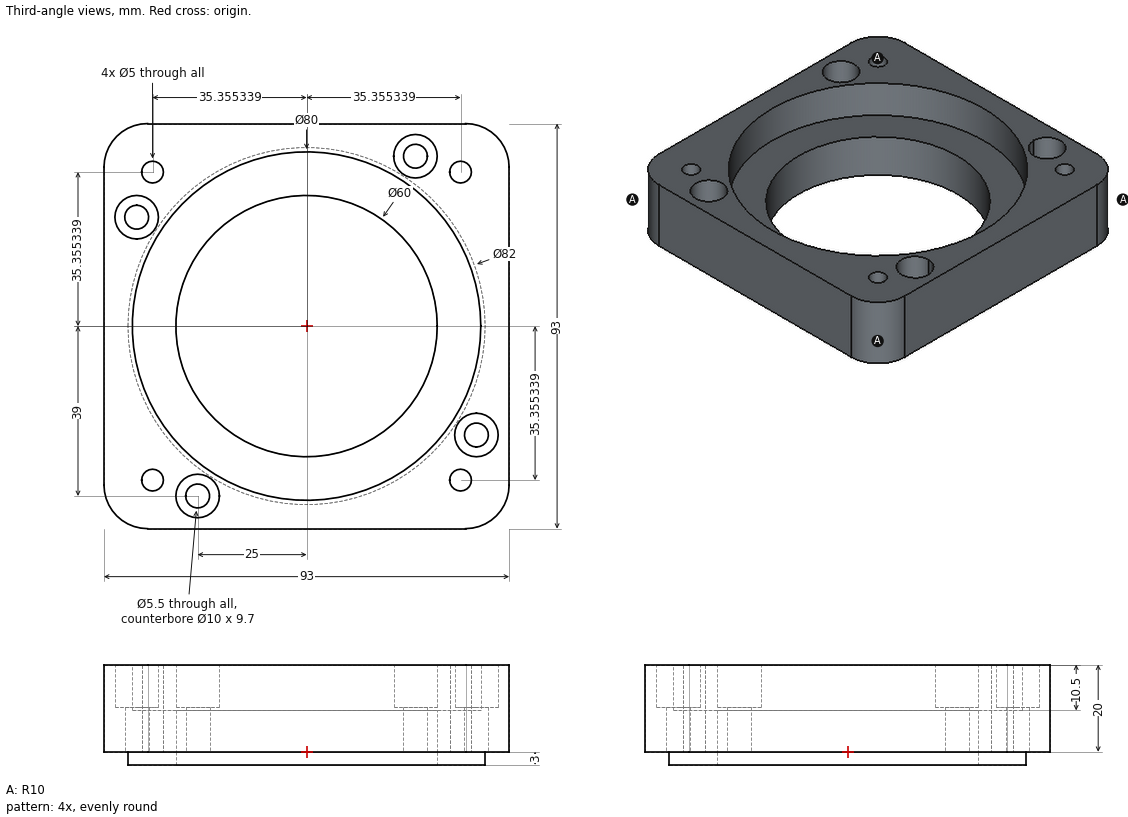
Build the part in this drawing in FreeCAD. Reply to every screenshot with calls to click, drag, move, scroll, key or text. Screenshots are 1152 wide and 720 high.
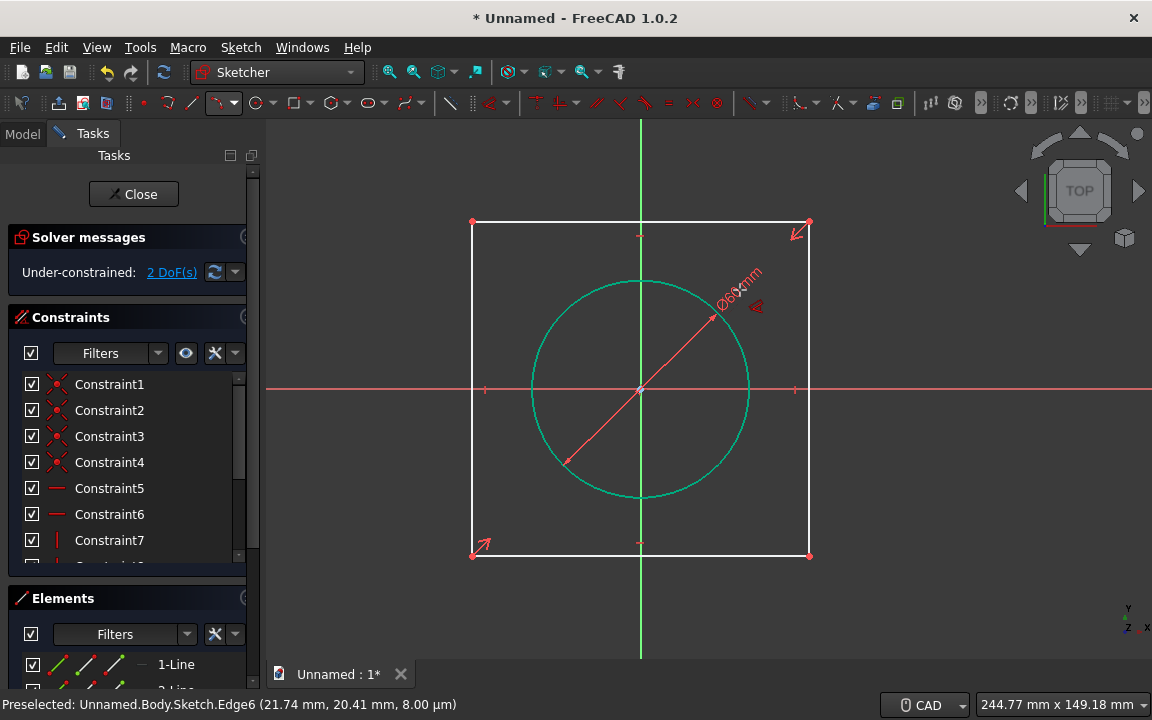
click(573, 556)
click(563, 590)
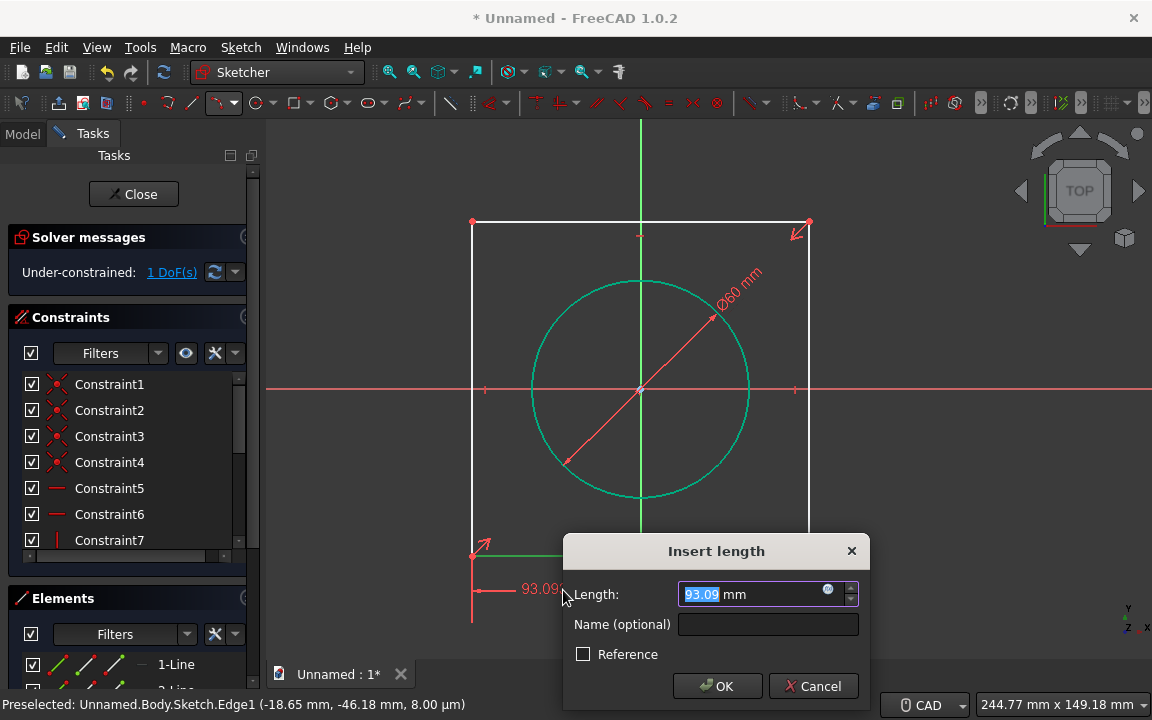
text(93)
key(Return)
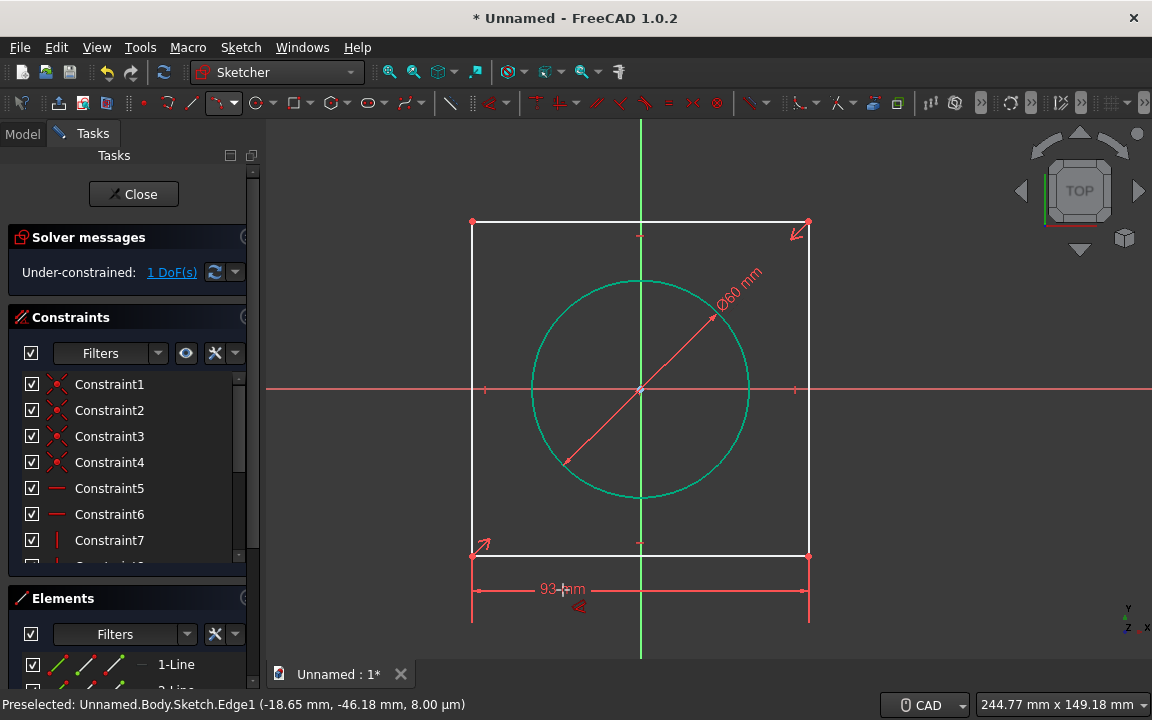
click(809, 456)
click(843, 312)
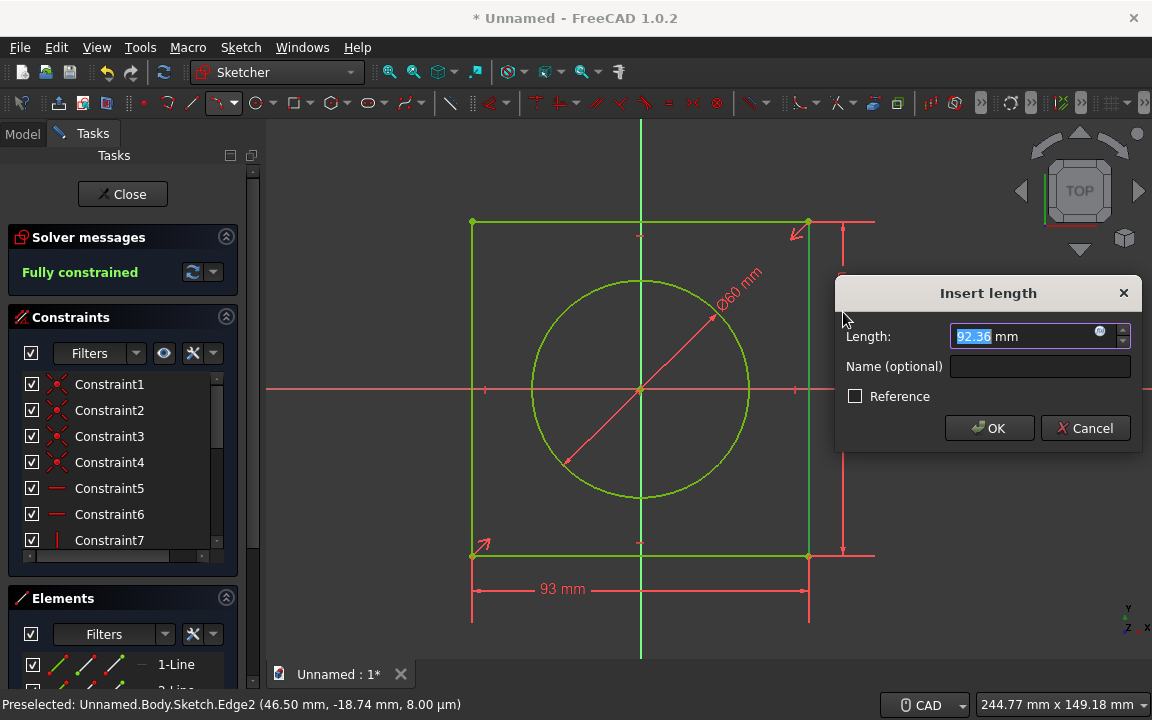
text(93)
key(Return)
key(Escape)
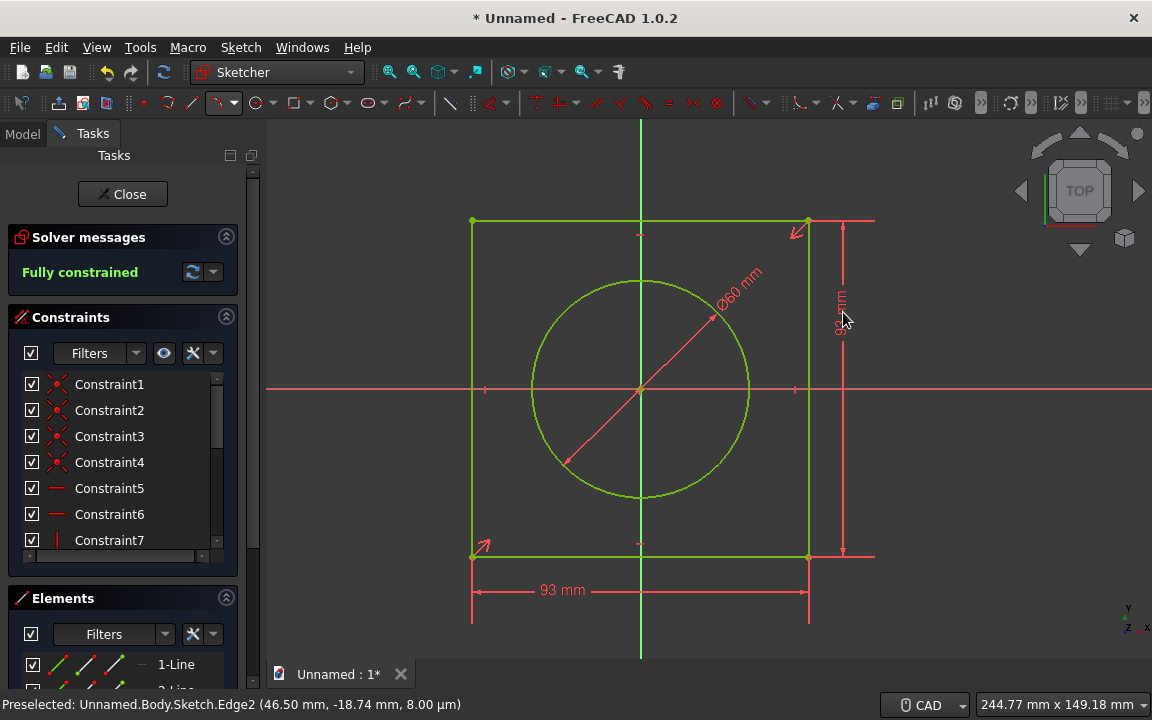
click(123, 194)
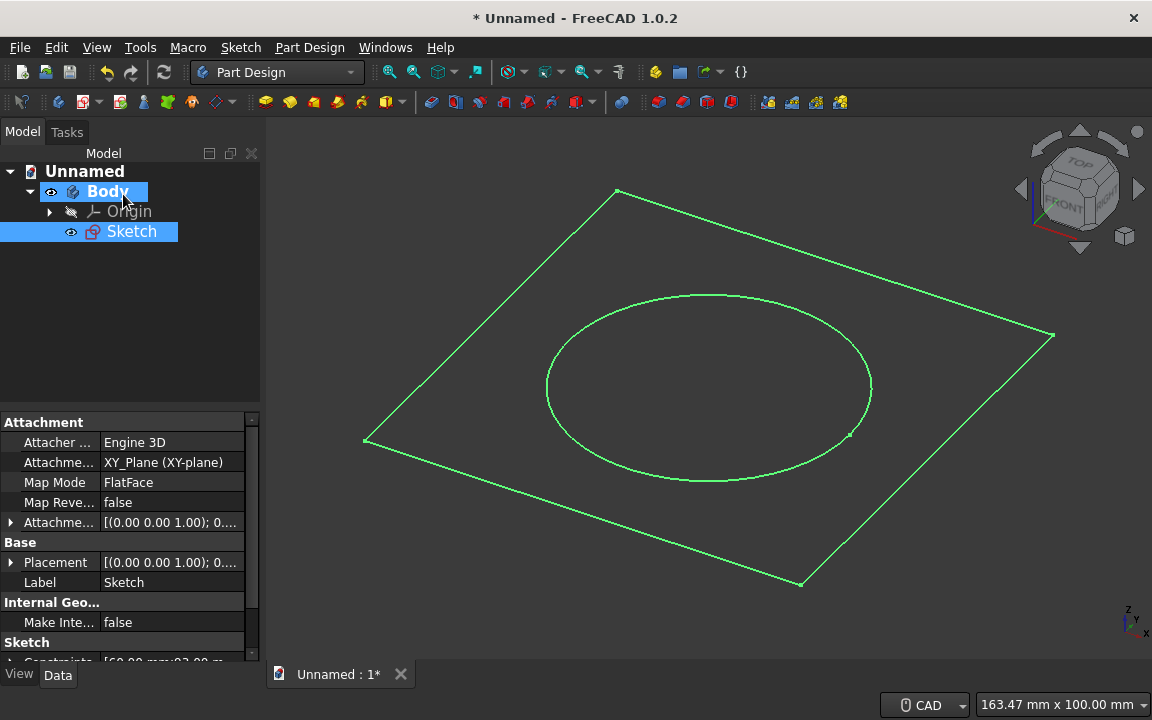
click(266, 102)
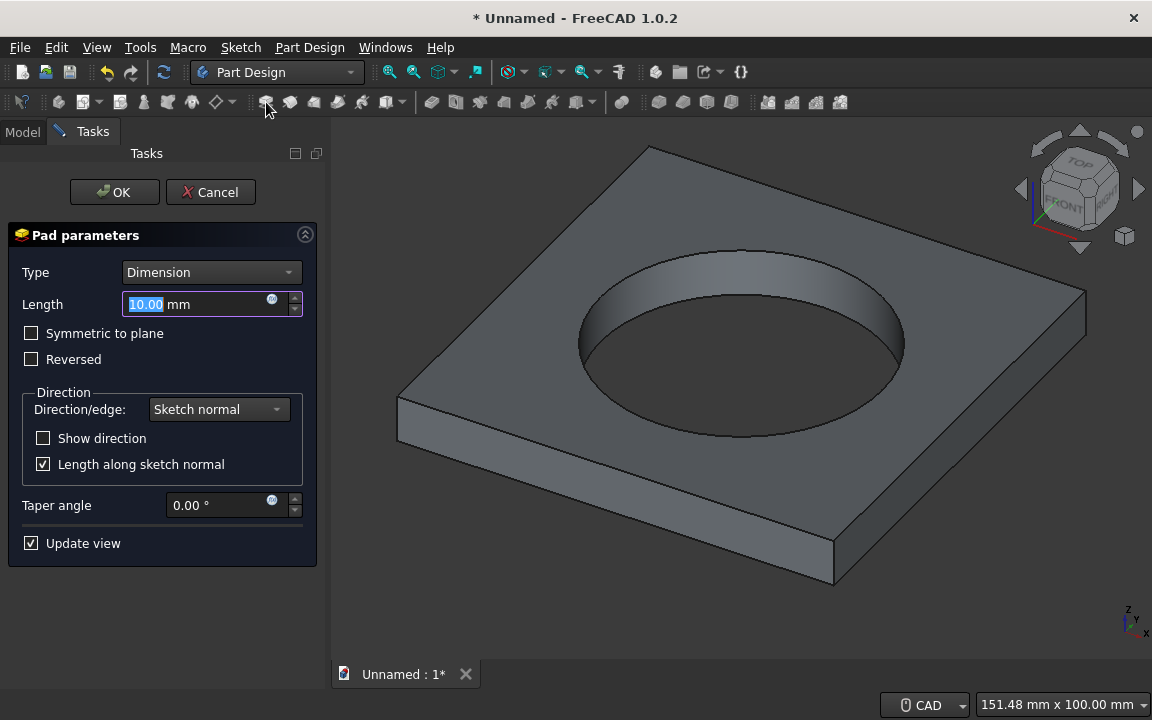
text(20)
key(Tab)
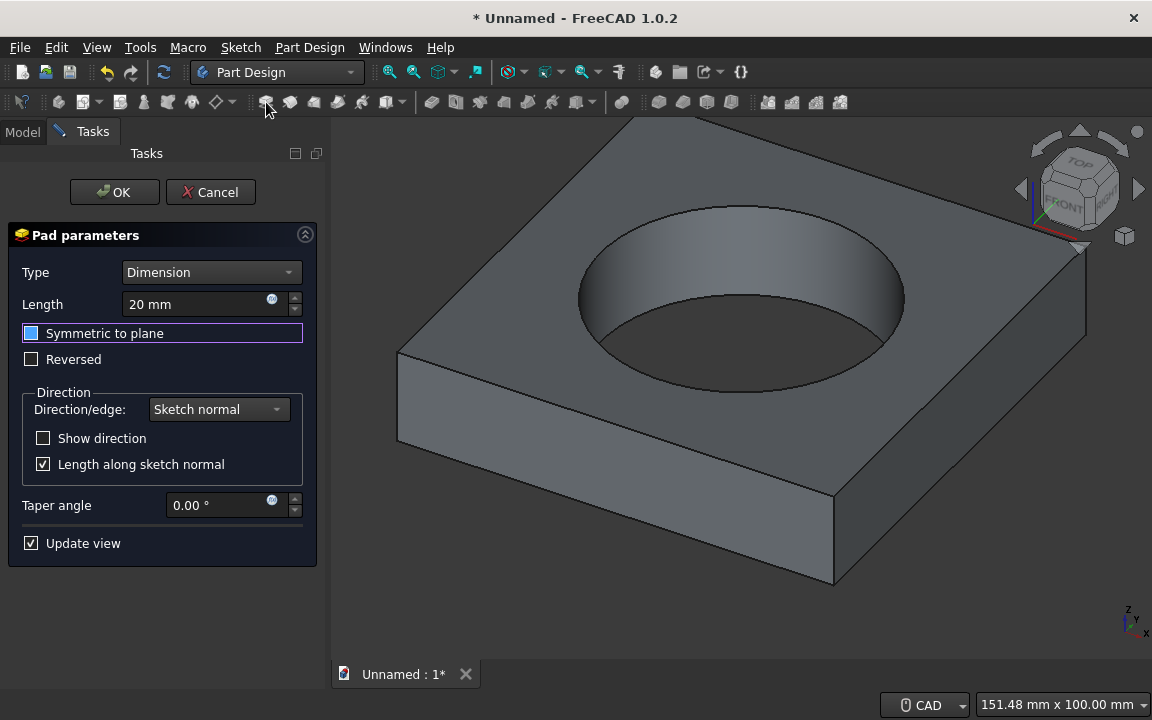
click(115, 192)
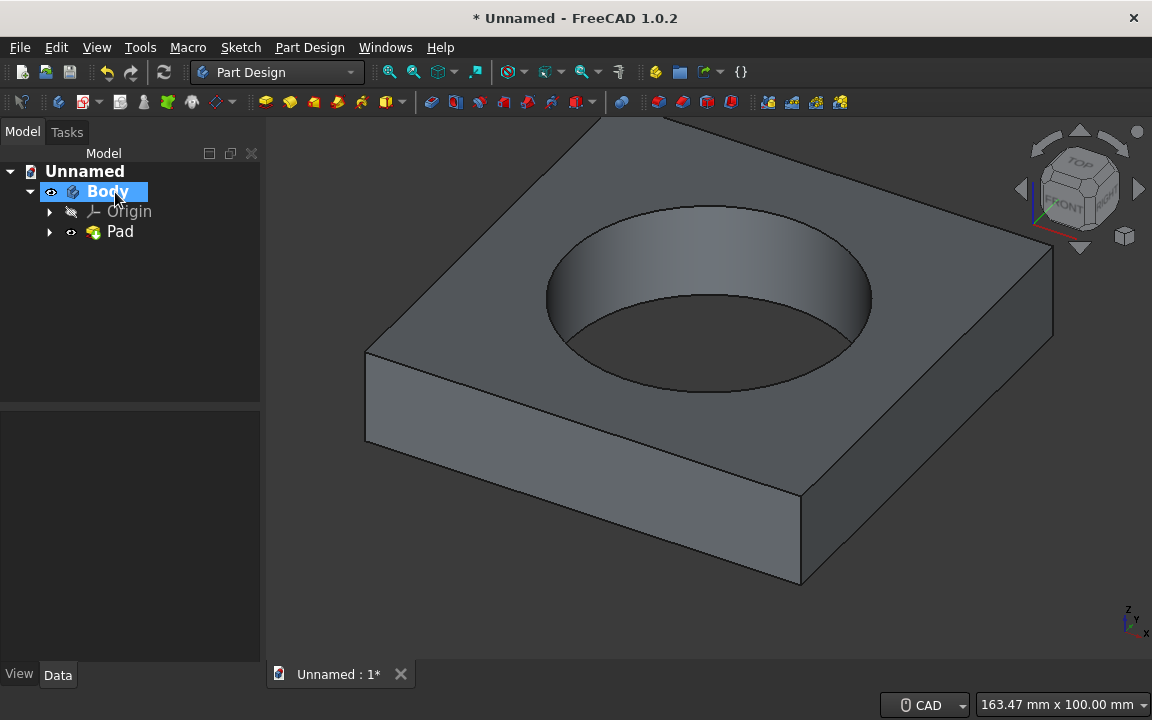
click(390, 72)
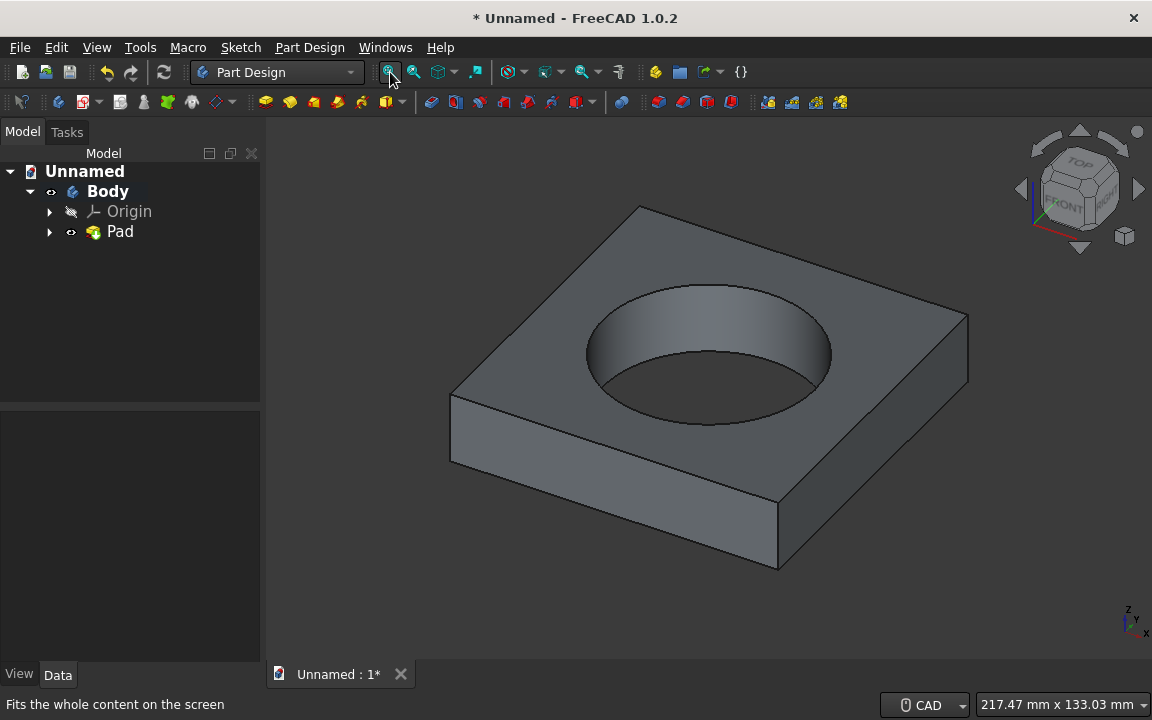
click(778, 535)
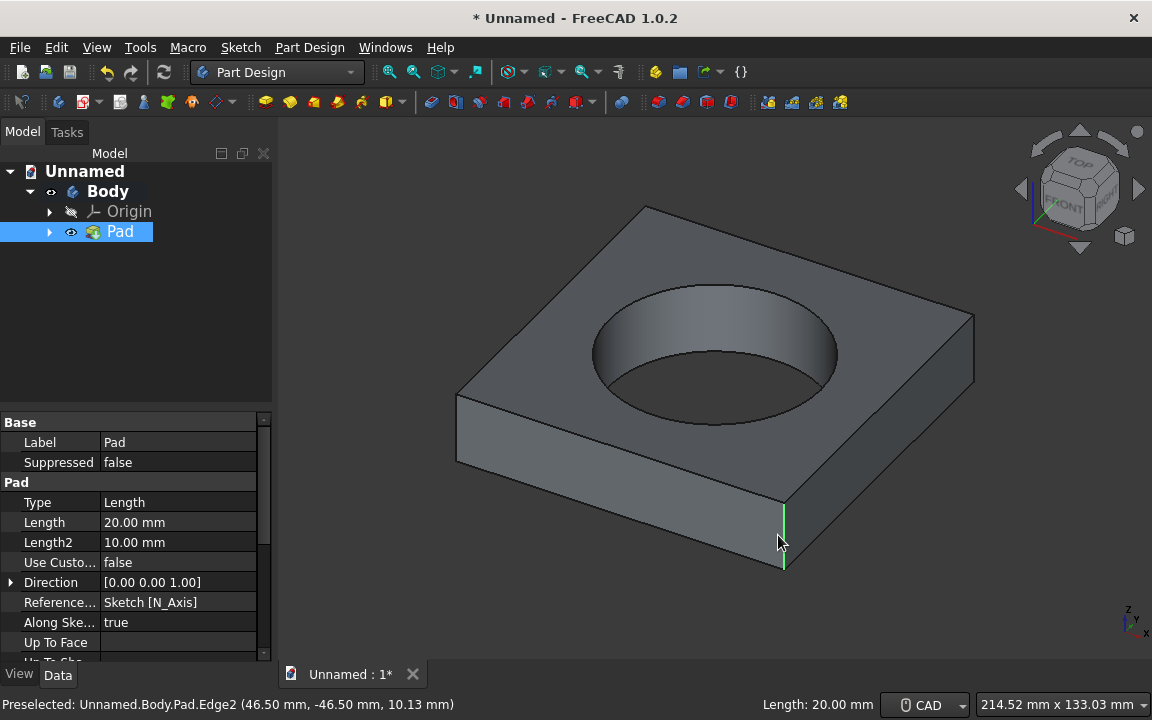
key(0)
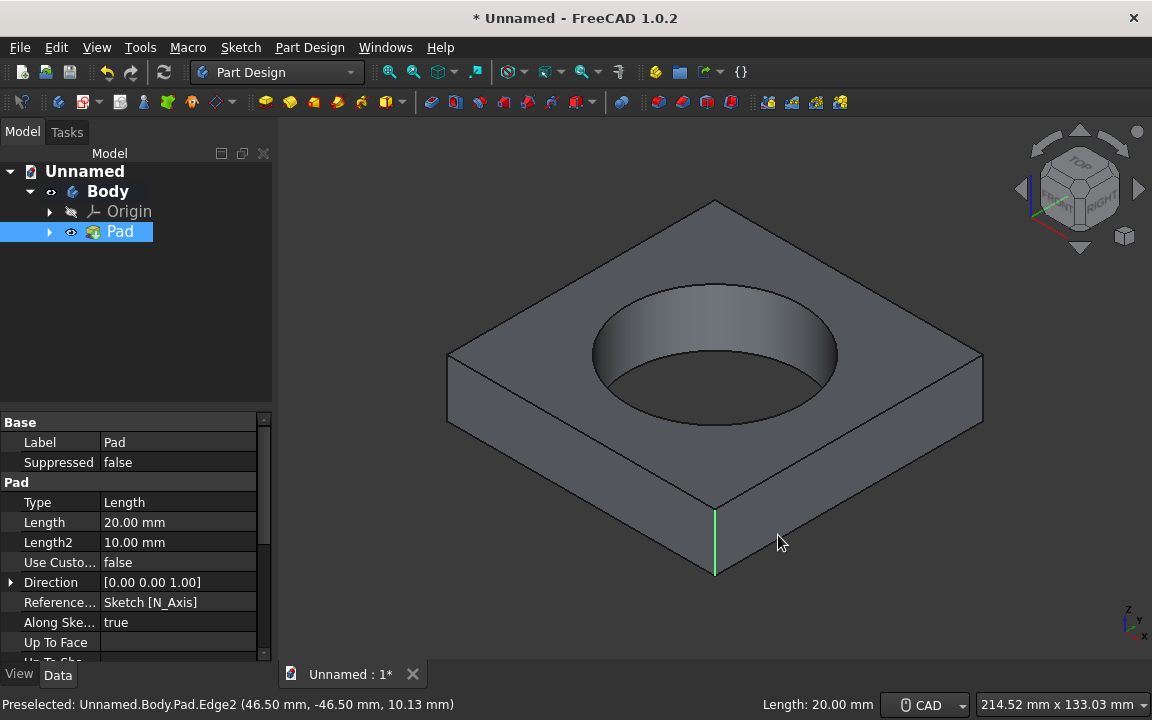
key(2)